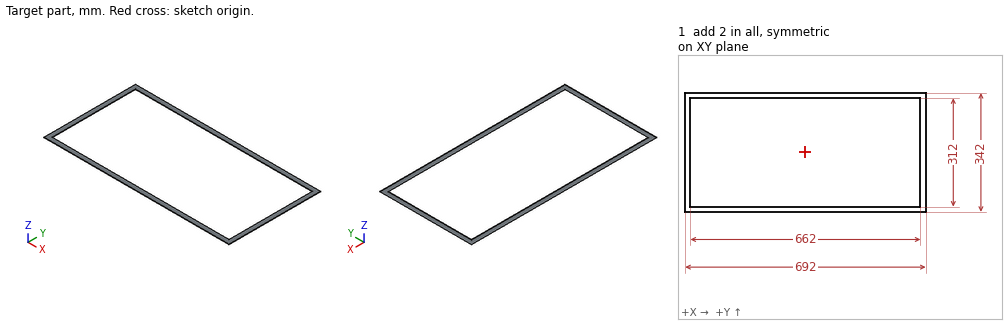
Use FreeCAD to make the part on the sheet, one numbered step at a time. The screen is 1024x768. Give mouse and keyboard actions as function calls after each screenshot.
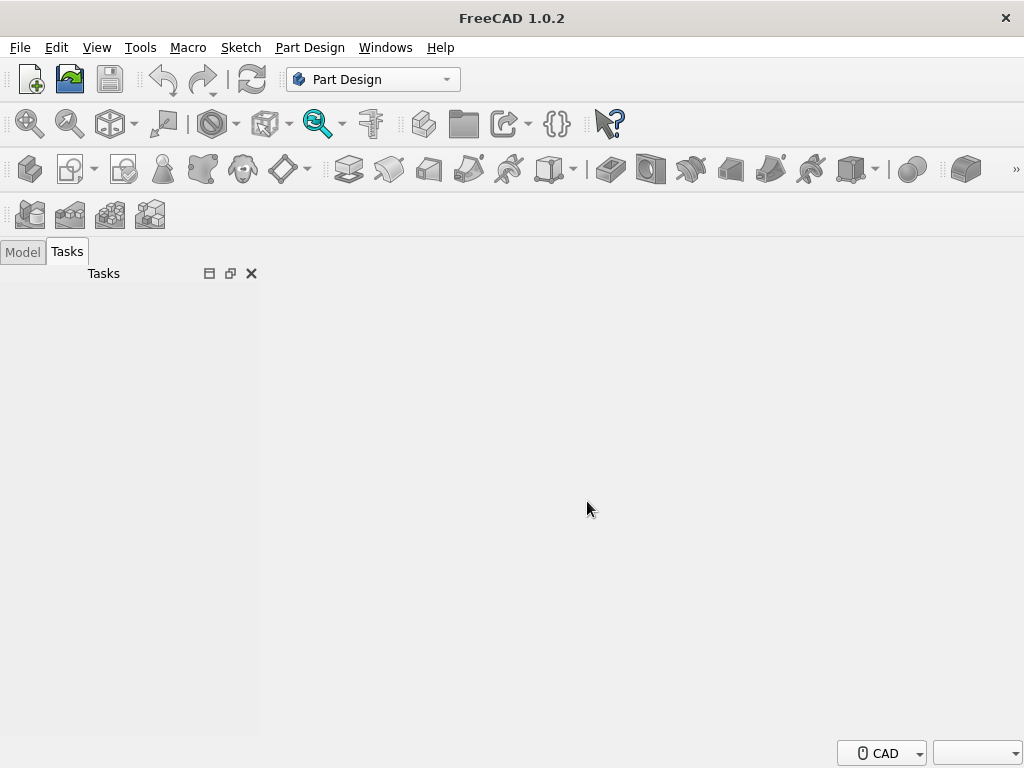
click(30, 80)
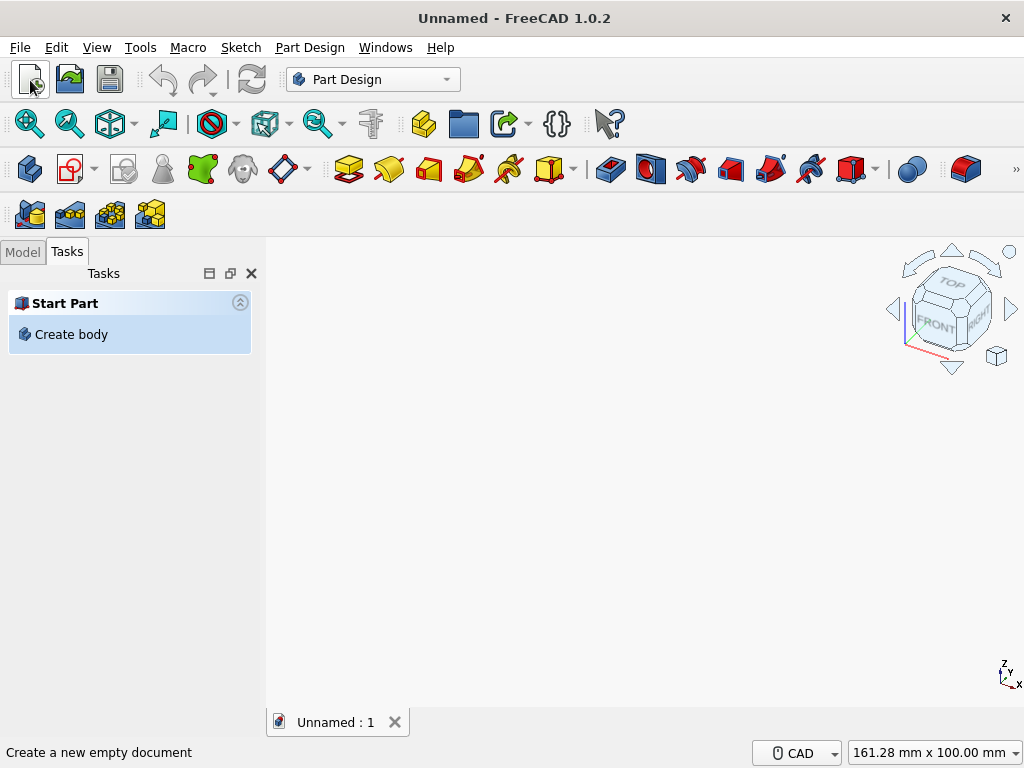
click(70, 170)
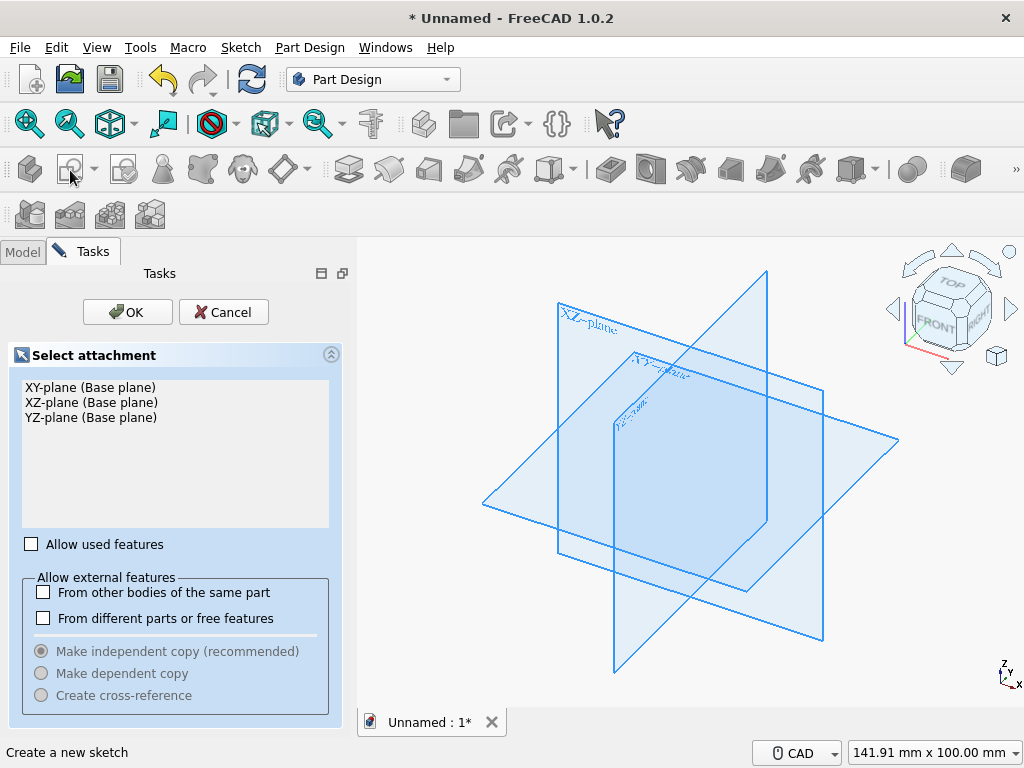
click(82, 388)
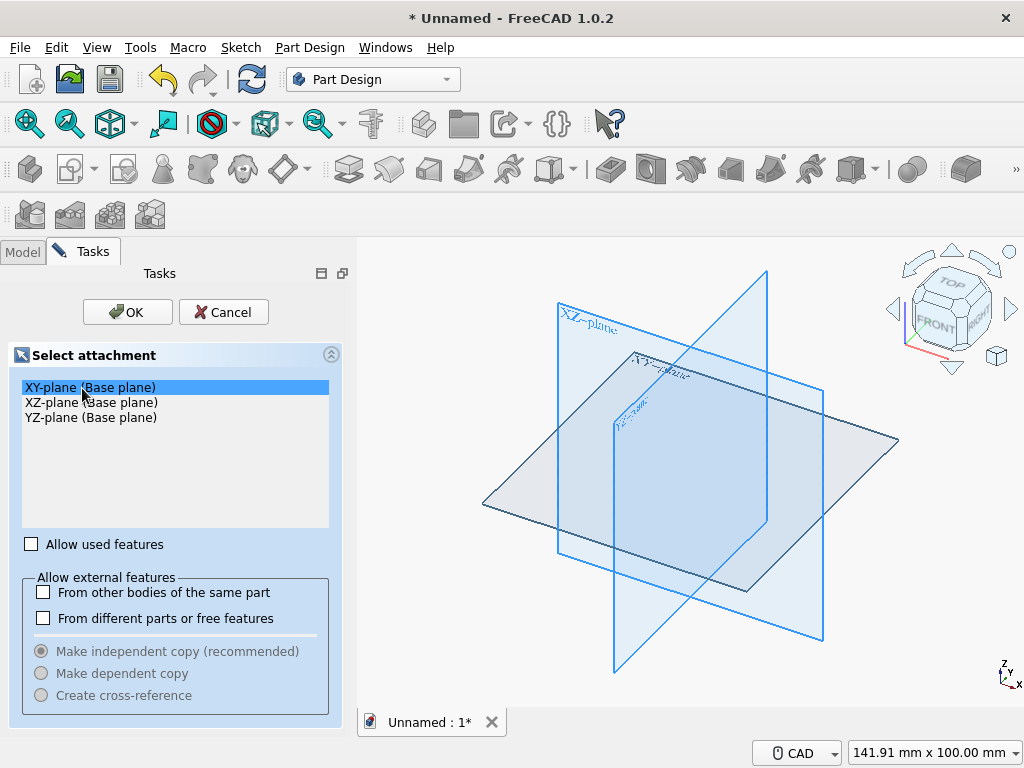
click(128, 312)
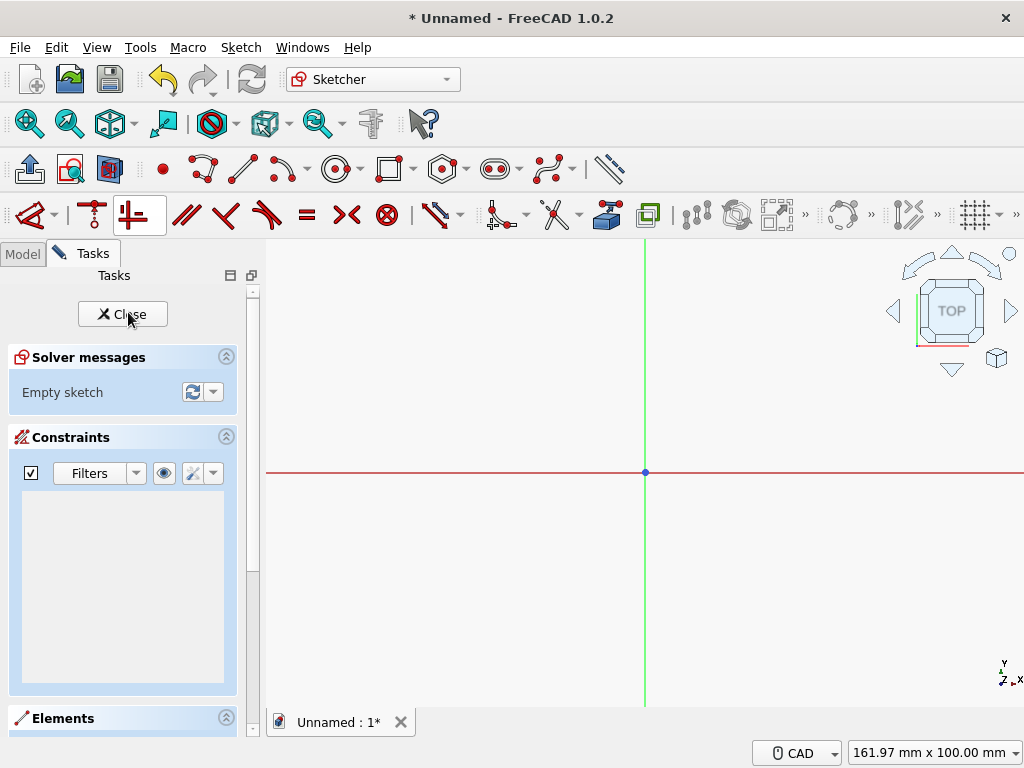
scroll(566, 473, down, 10)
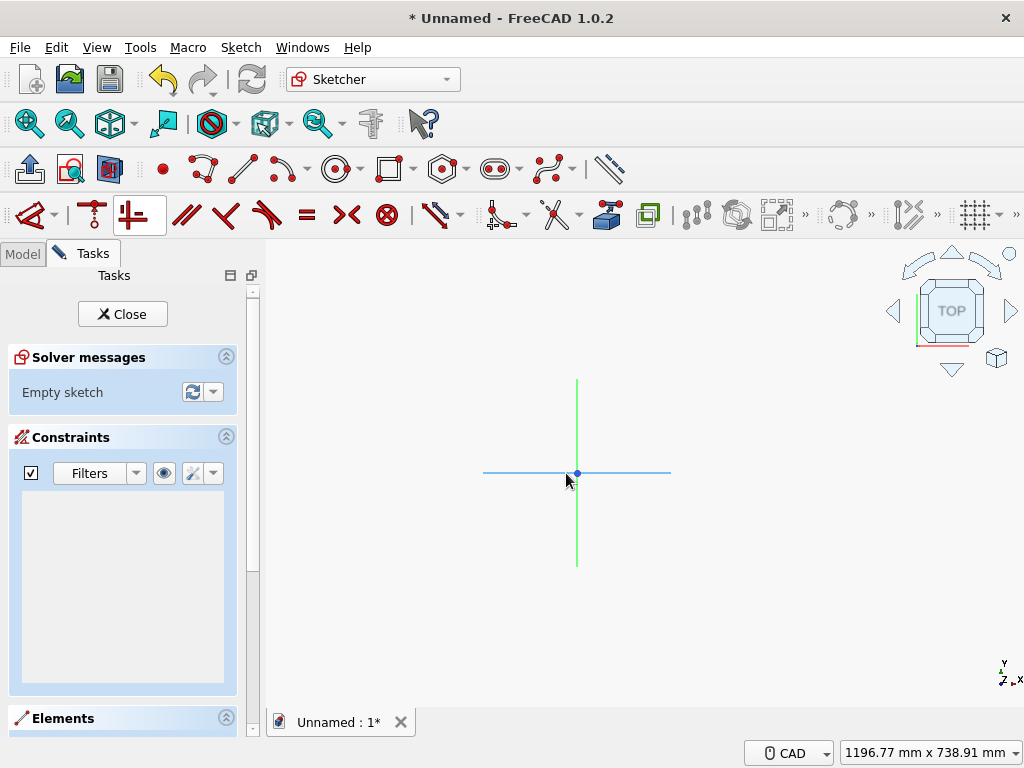
click(416, 170)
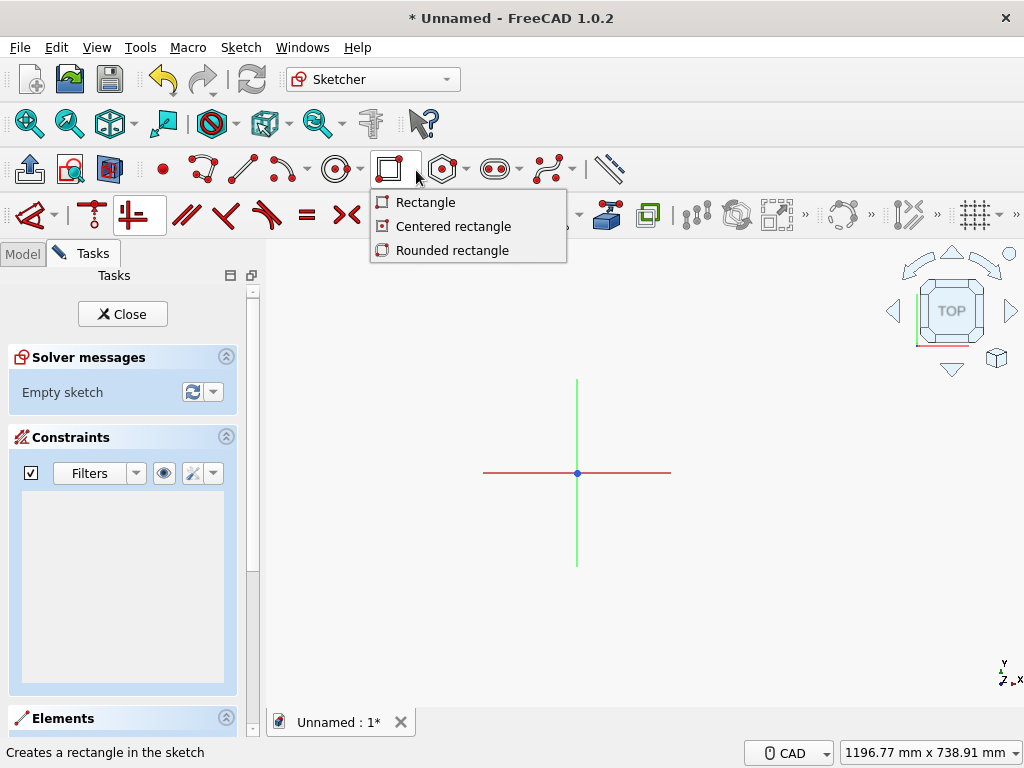
click(468, 226)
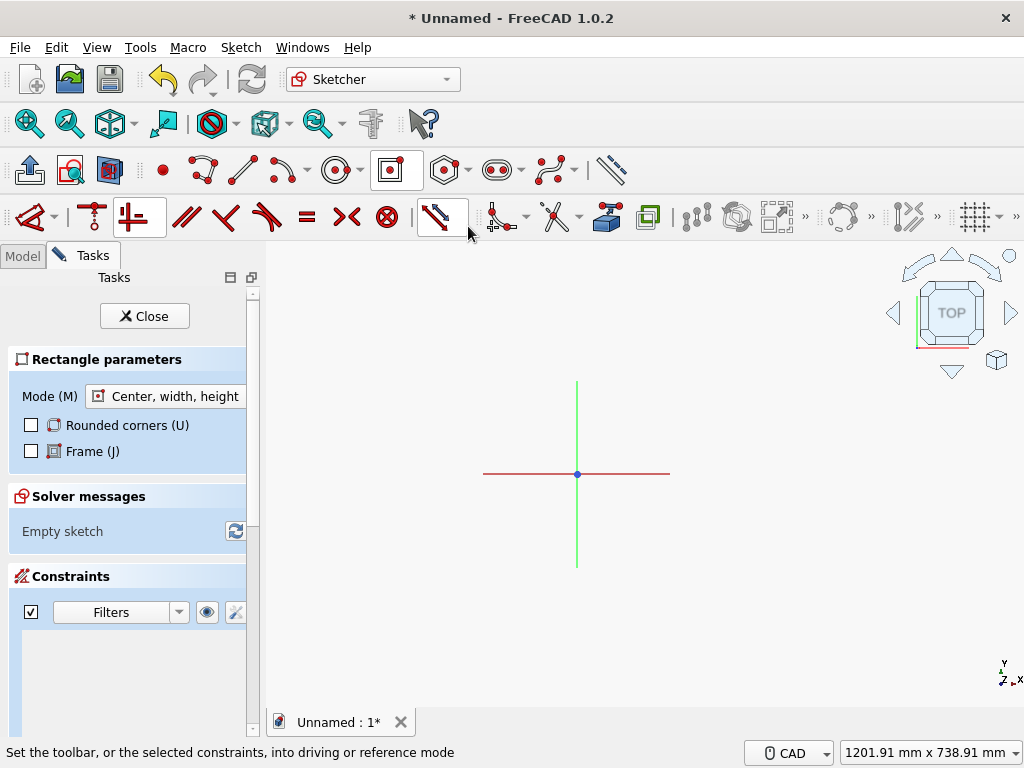
click(577, 474)
move(796, 367)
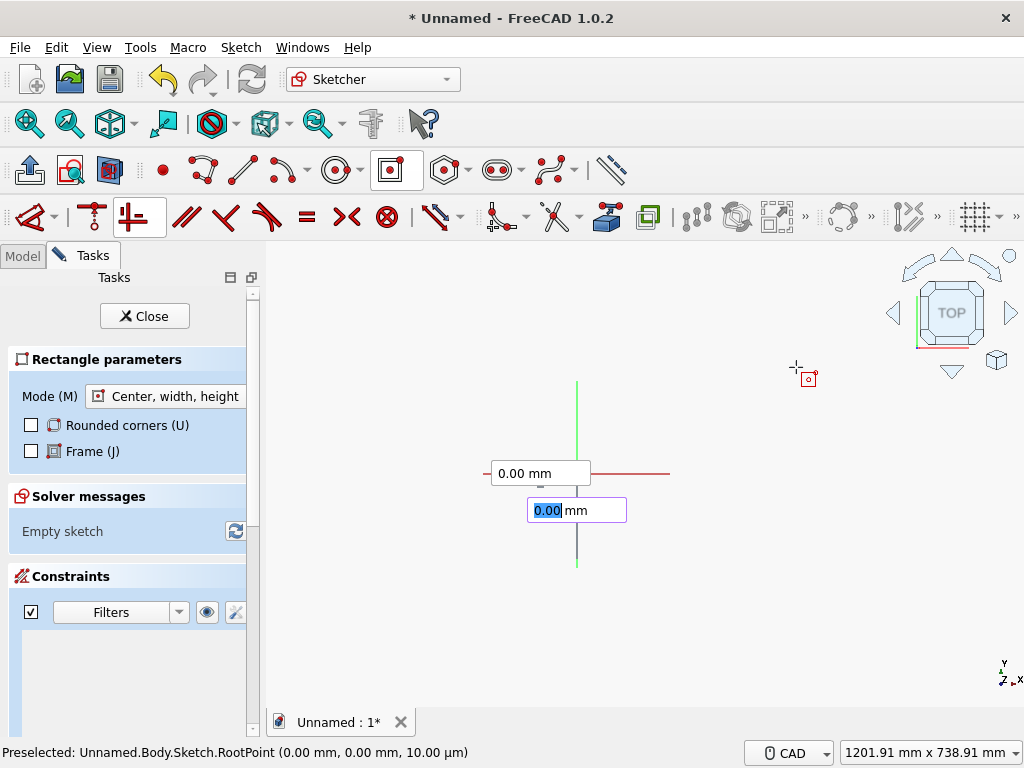
text(692)
key(Tab)
text(342)
key(Return)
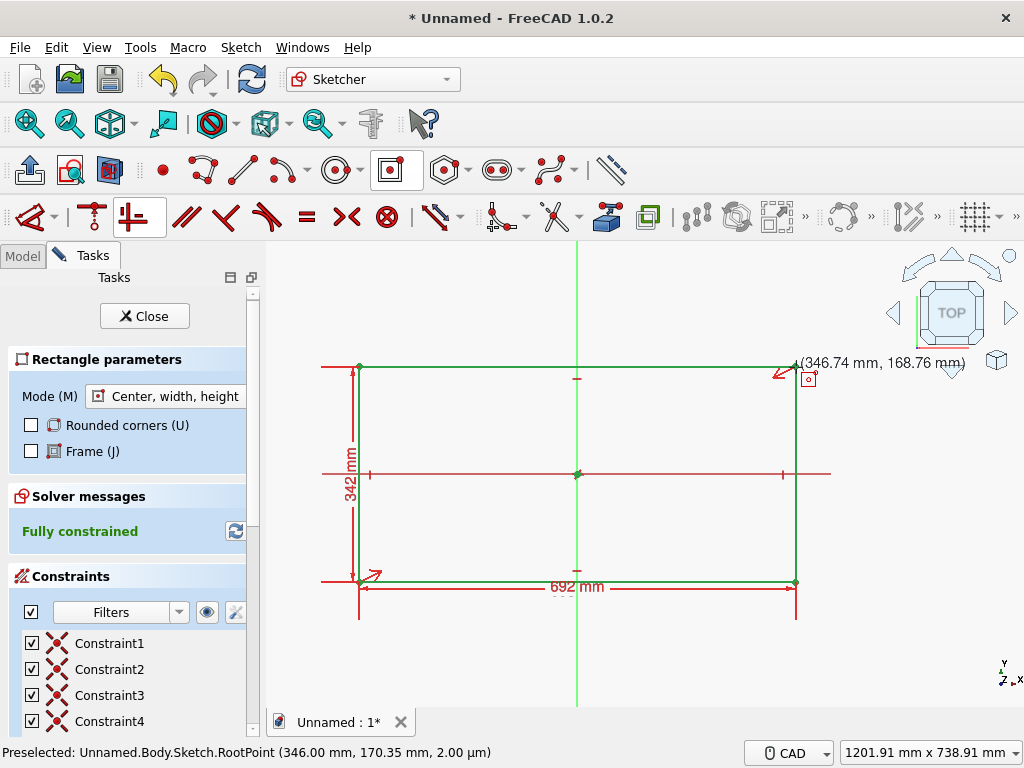
click(577, 474)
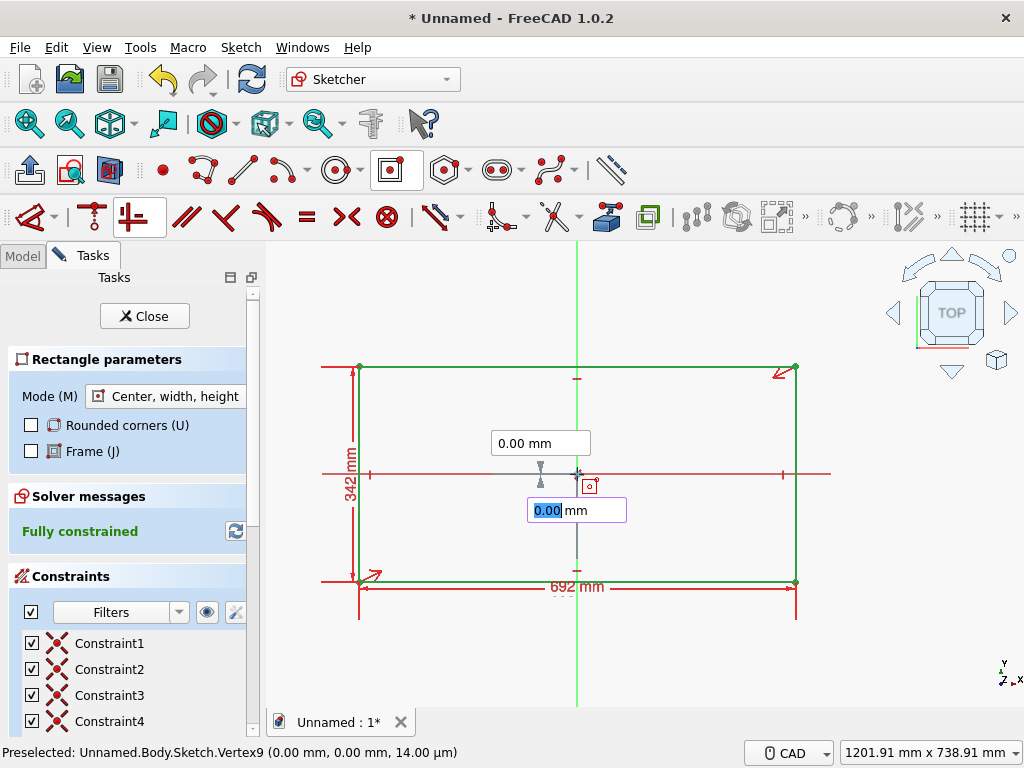
scroll(786, 376, up, 3)
move(786, 376)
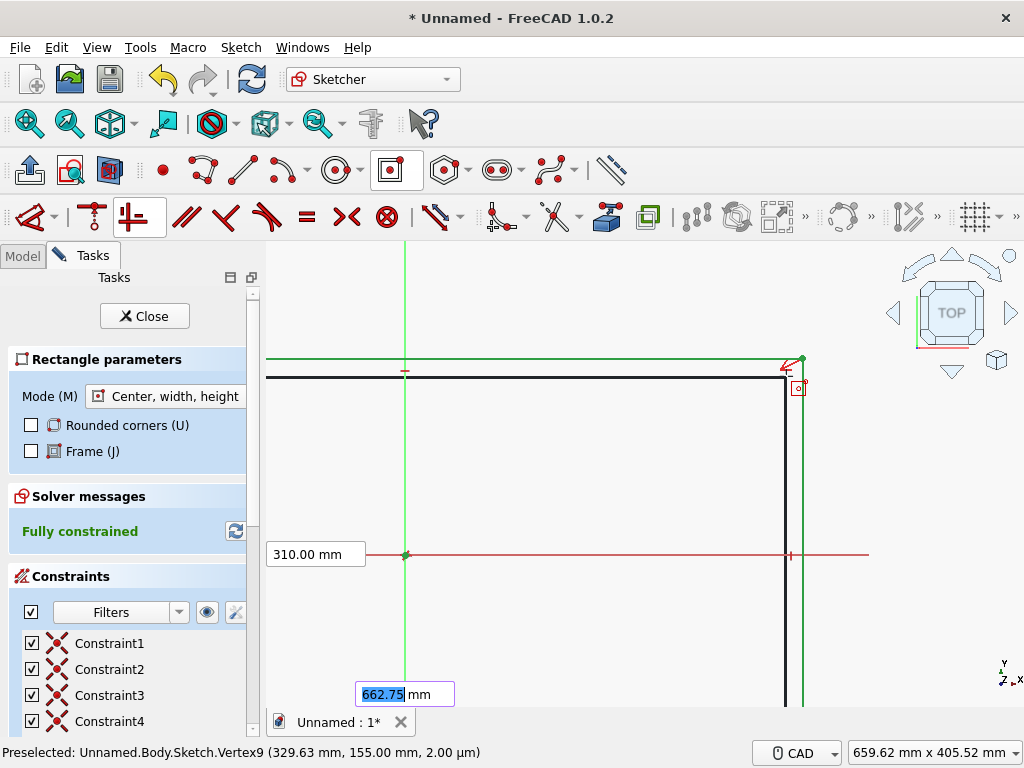
text(662)
key(Tab)
text(312)
key(Return)
key(Escape)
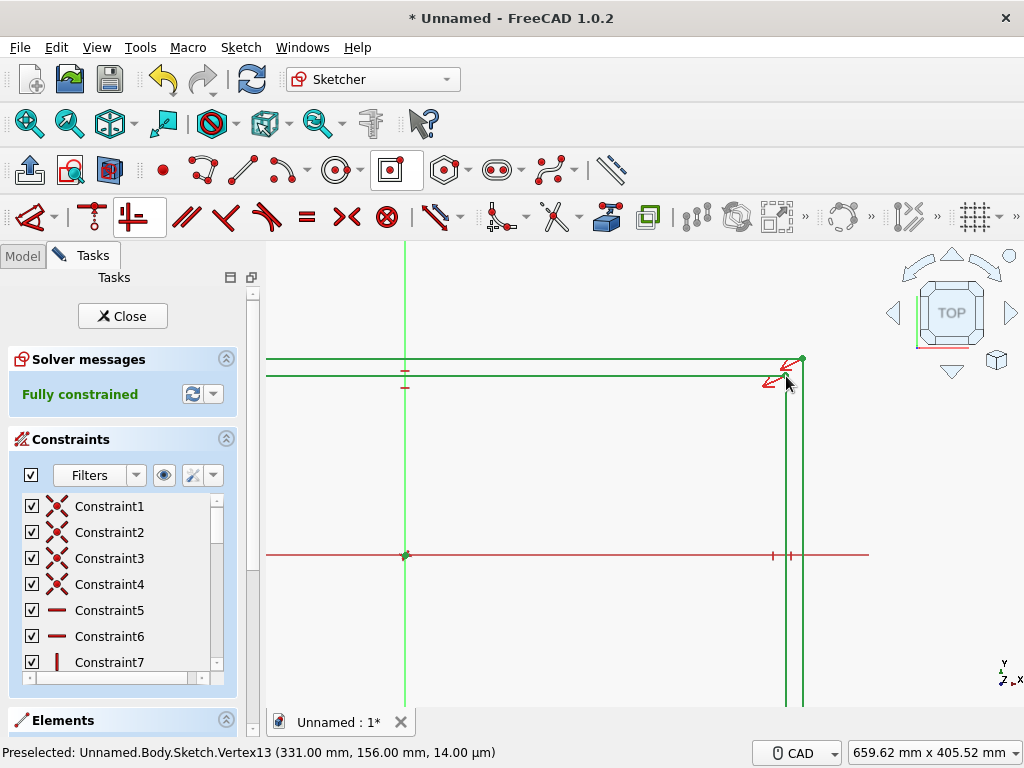
click(123, 316)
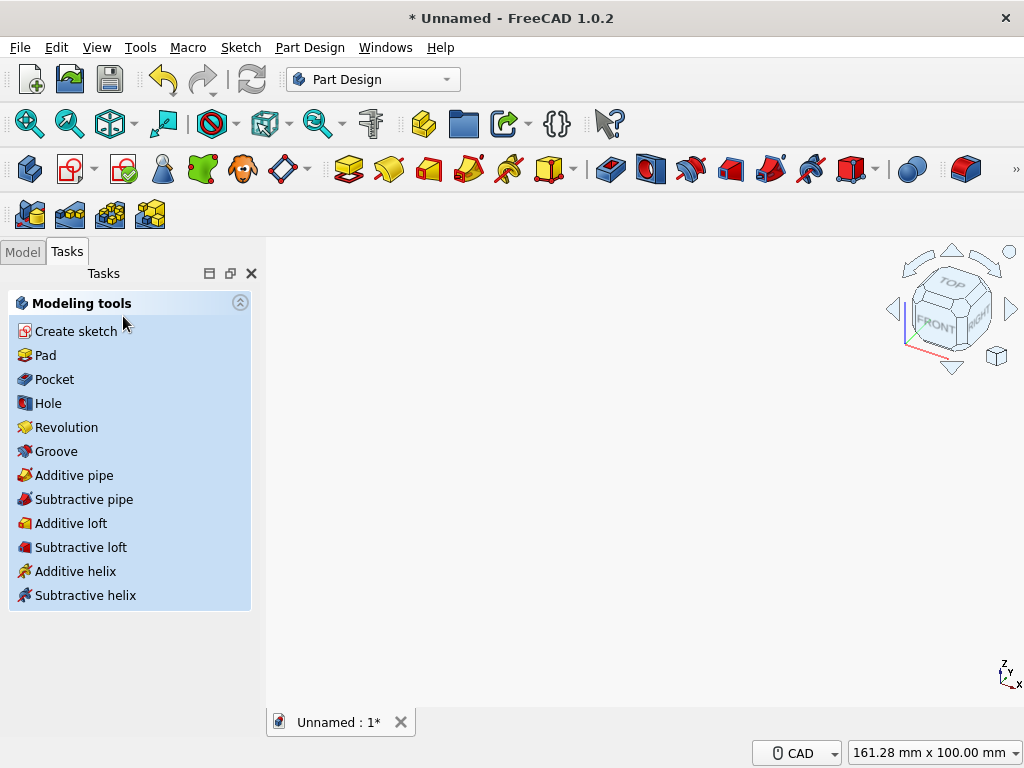
click(350, 170)